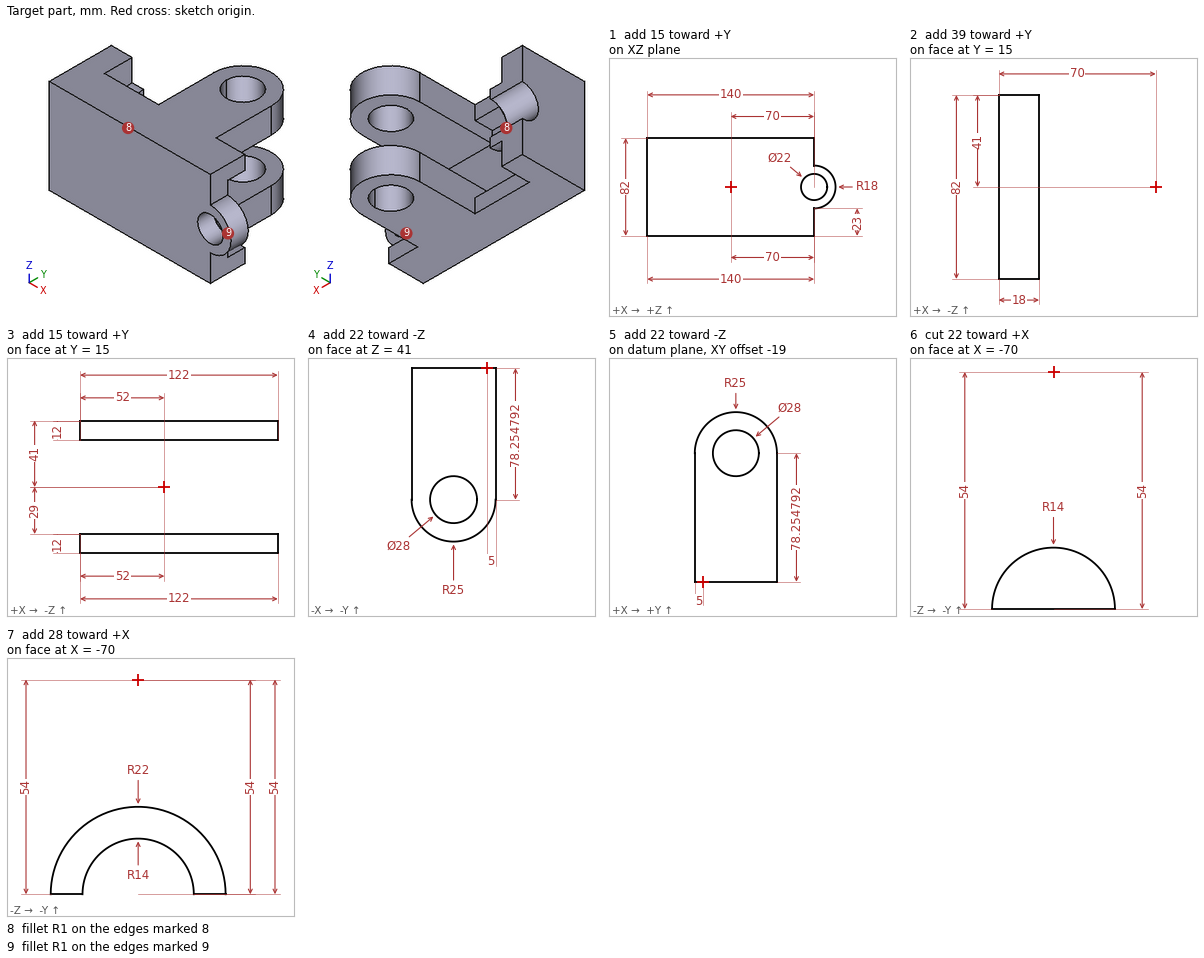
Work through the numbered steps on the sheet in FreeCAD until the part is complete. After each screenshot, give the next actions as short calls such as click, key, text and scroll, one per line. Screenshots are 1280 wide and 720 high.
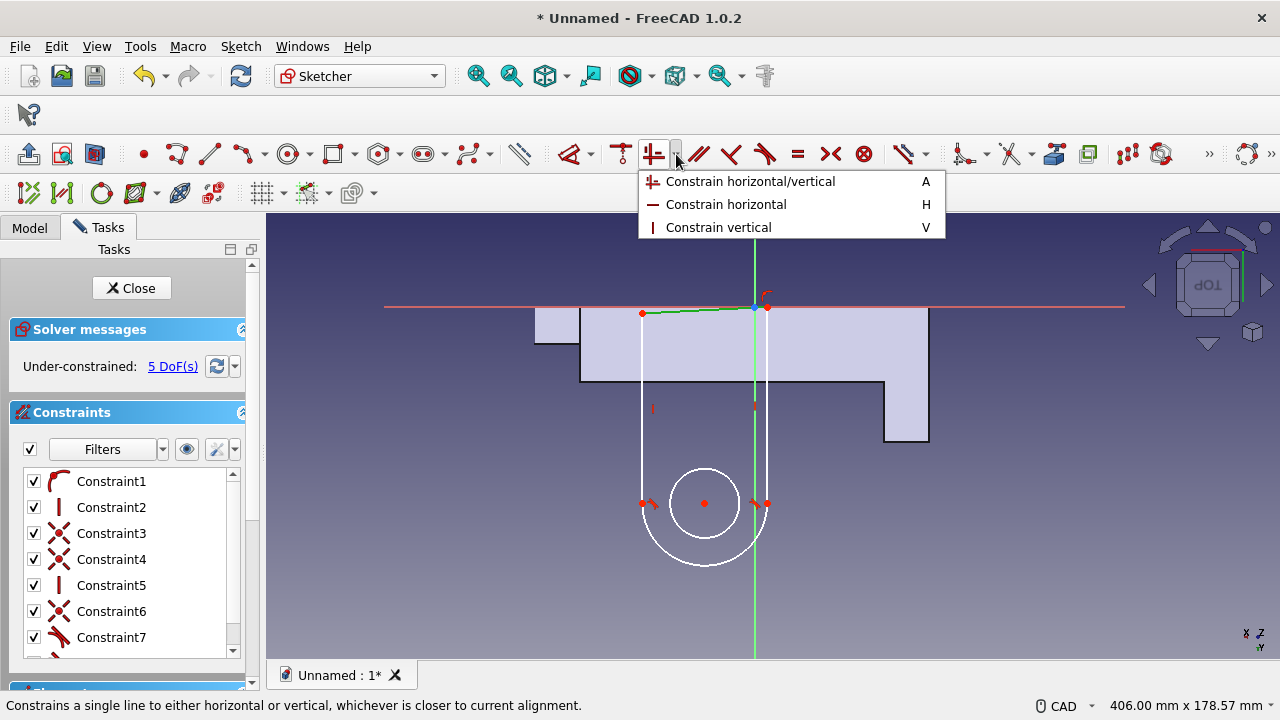
click(792, 204)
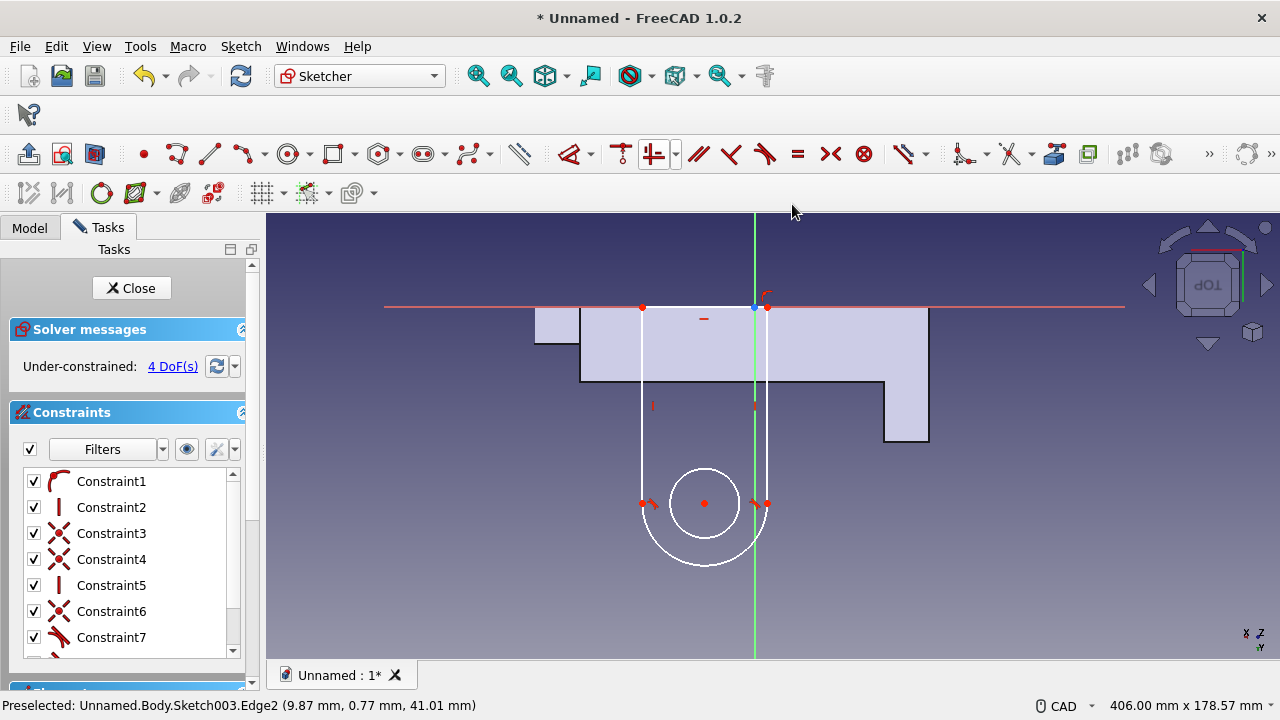
click(568, 154)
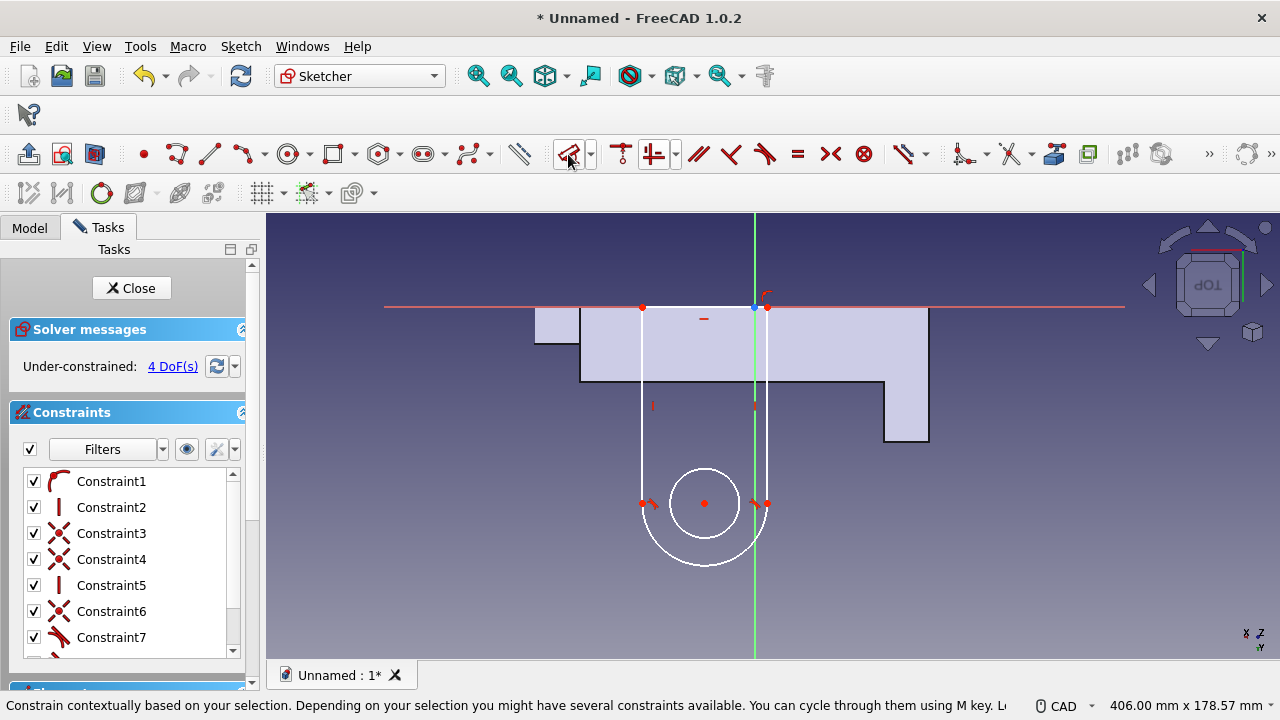
click(668, 554)
click(649, 580)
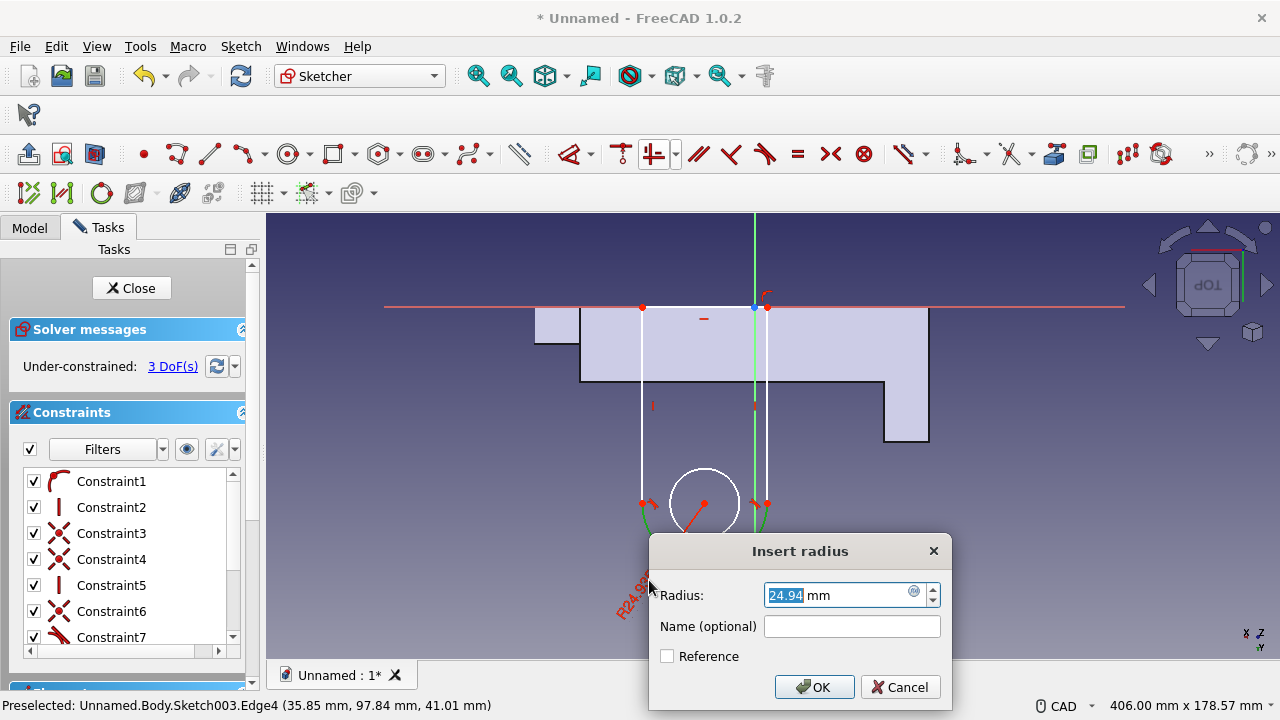
text(25)
key(Return)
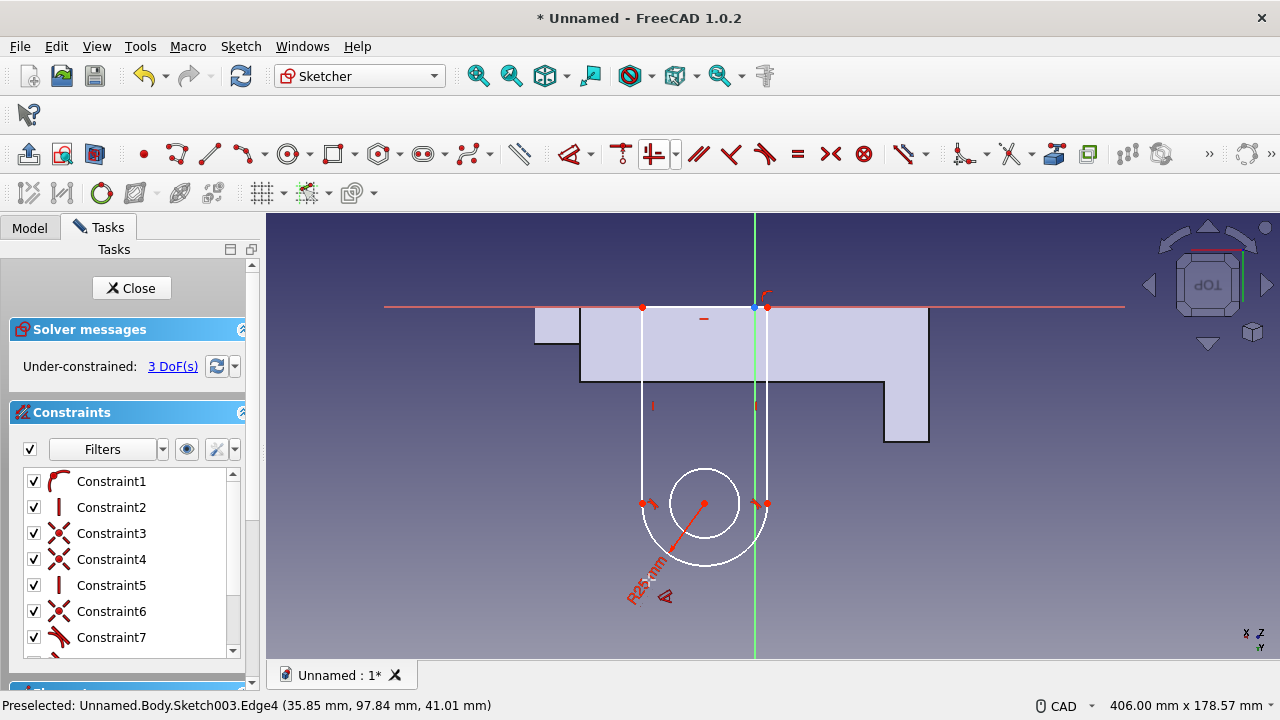
click(729, 479)
click(723, 440)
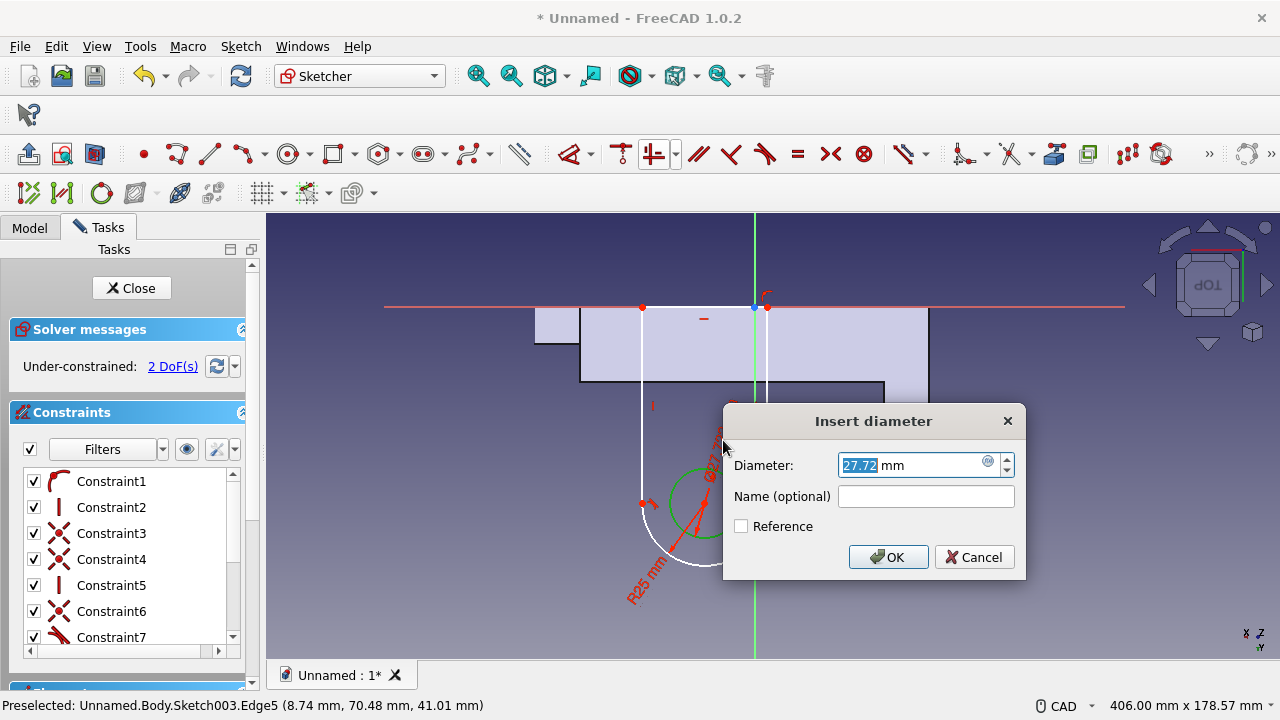
text(28)
key(Return)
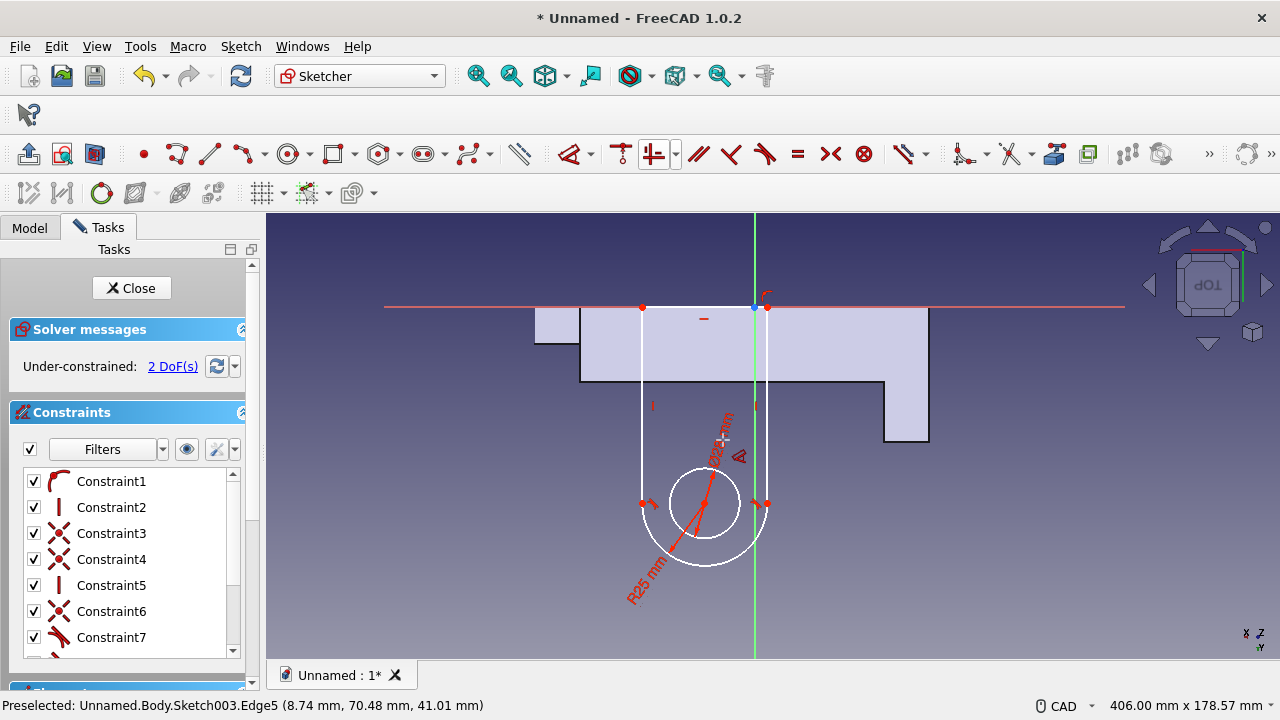
scroll(767, 503, up, 6)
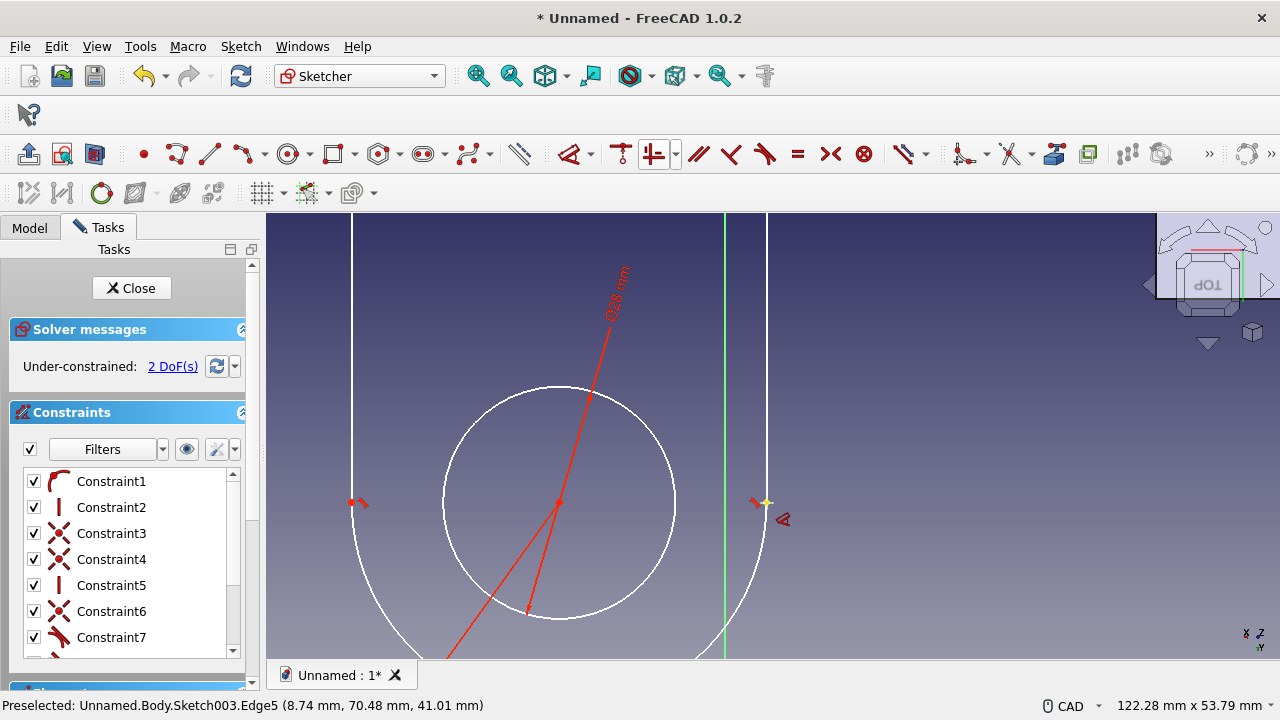
click(767, 503)
click(746, 537)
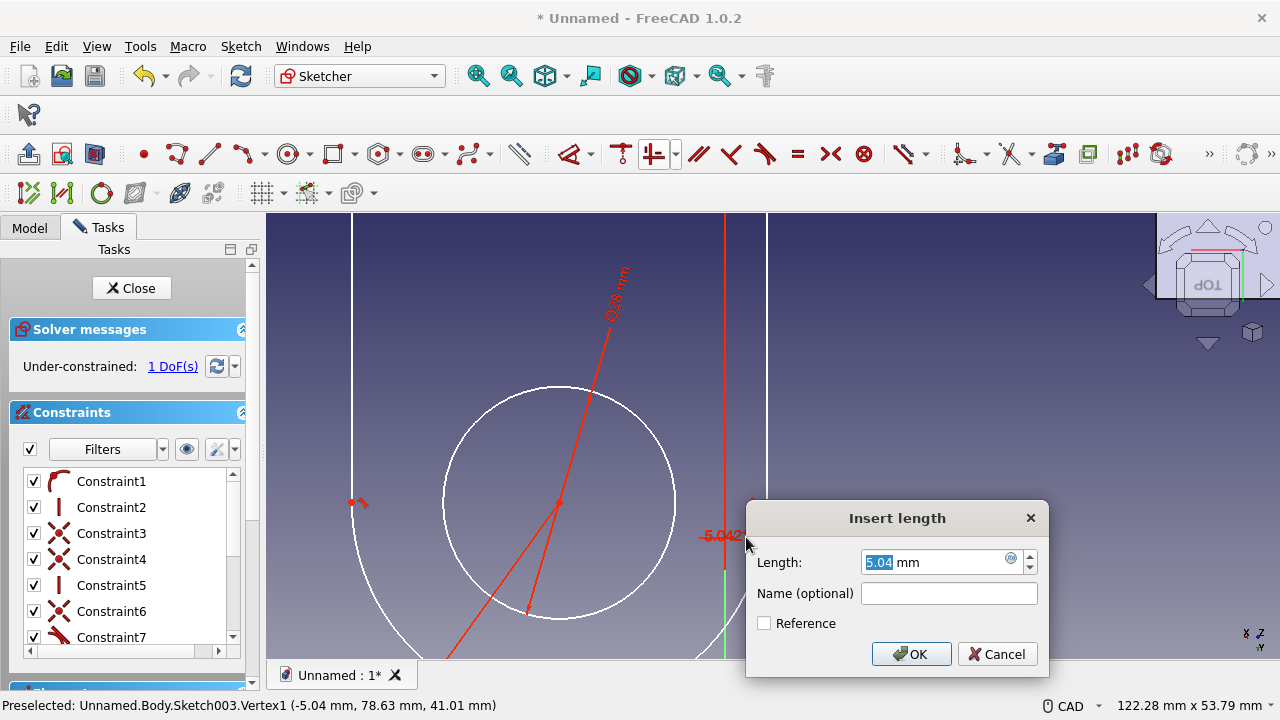
text(5)
key(Return)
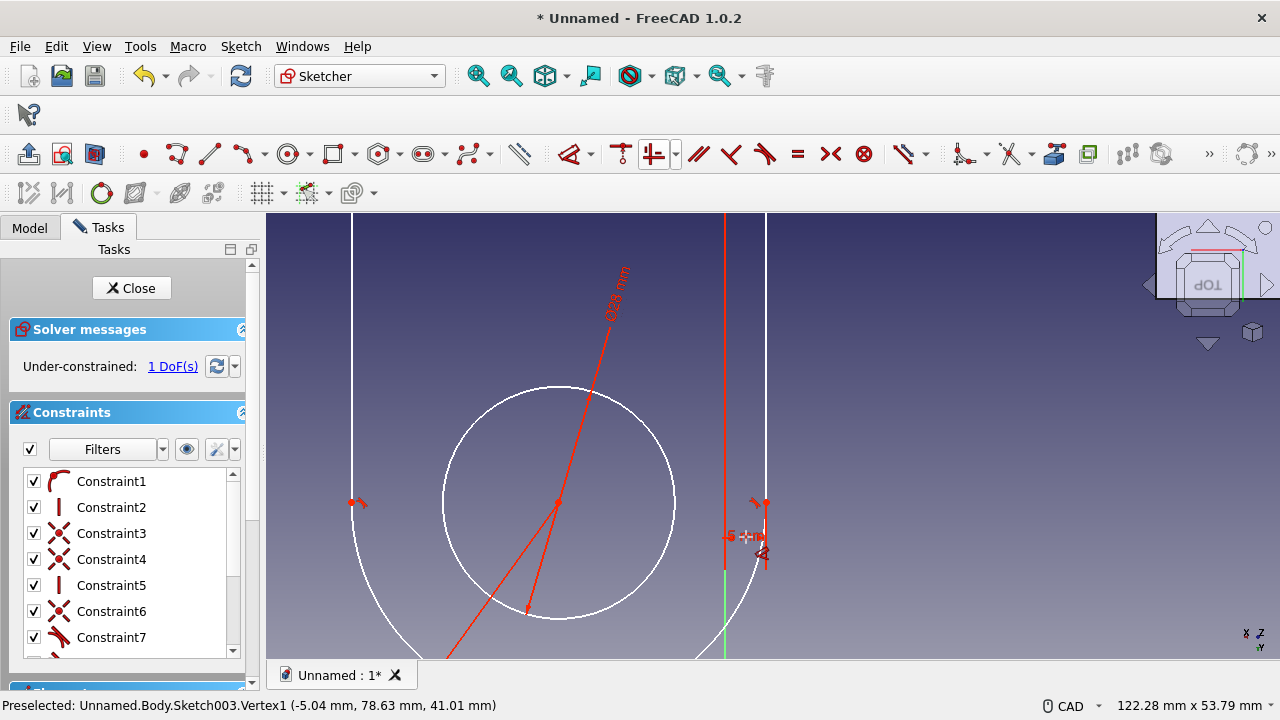
scroll(767, 504, down, 6)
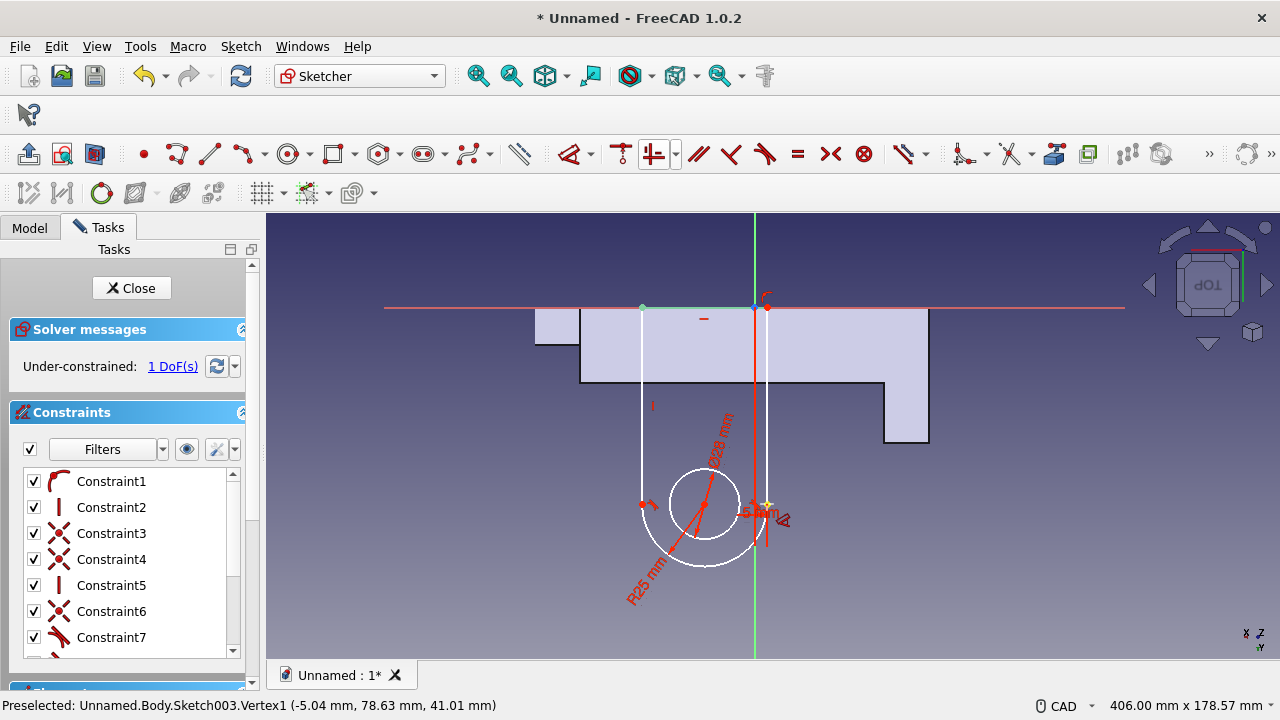
click(767, 445)
click(801, 406)